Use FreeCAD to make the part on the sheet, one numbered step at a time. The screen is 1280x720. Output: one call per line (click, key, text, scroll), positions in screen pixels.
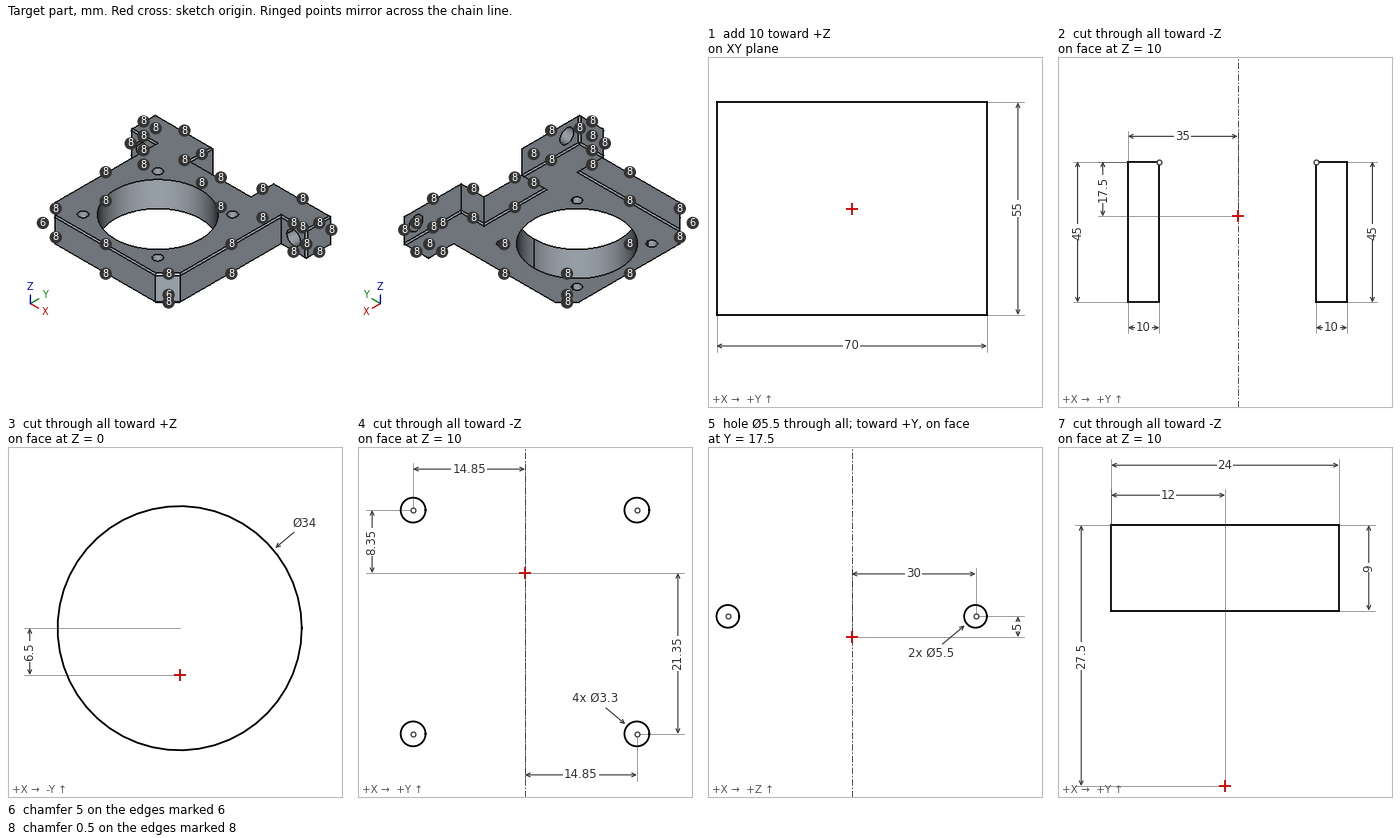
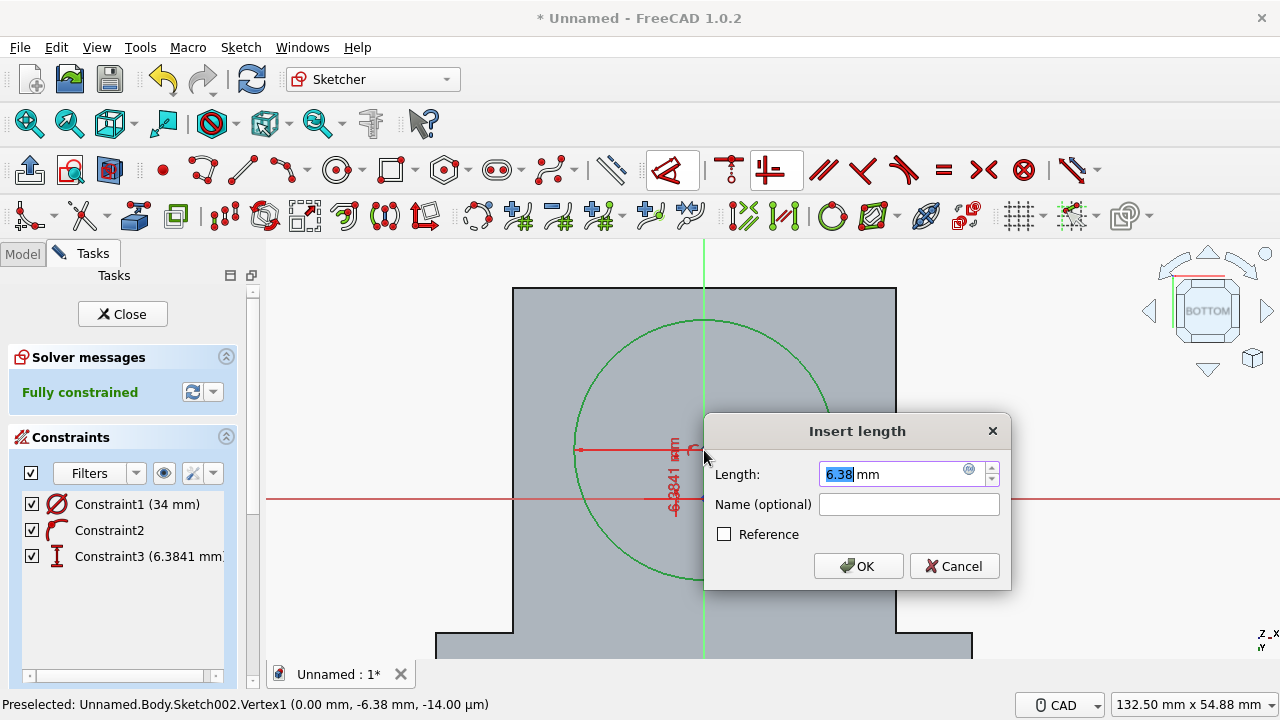
text(6.5)
key(Return)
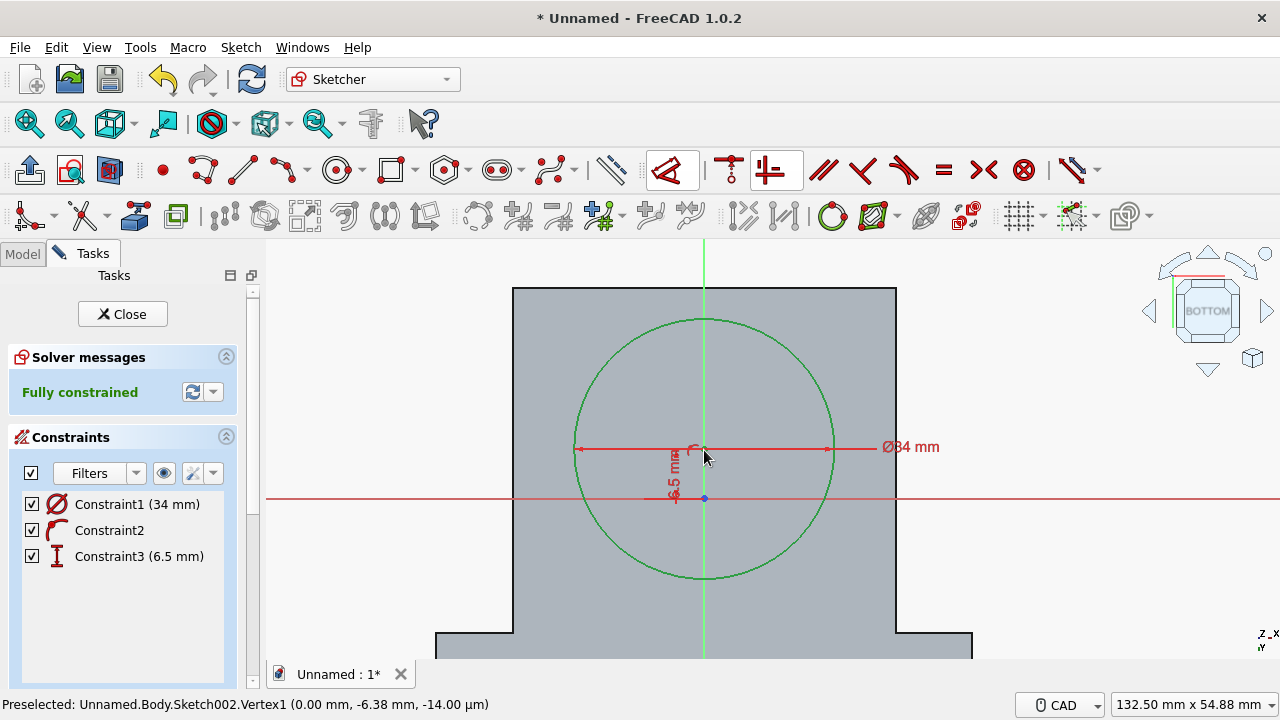
click(123, 314)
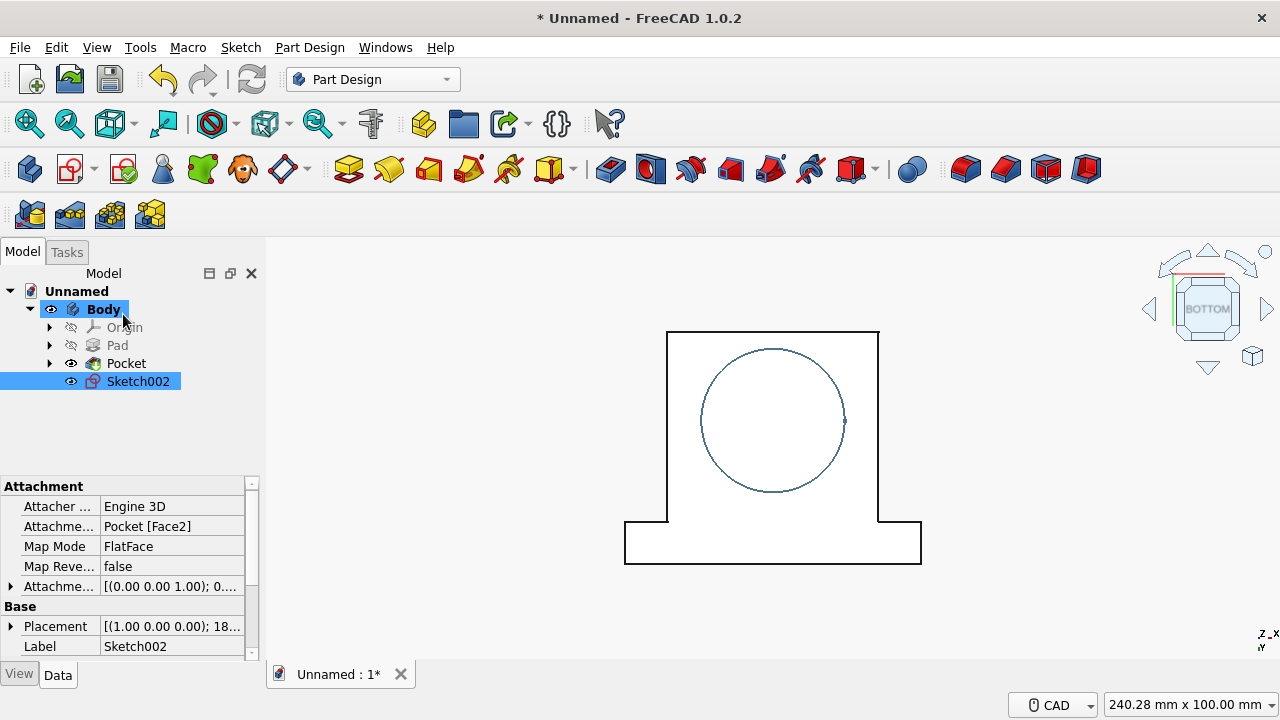
click(612, 170)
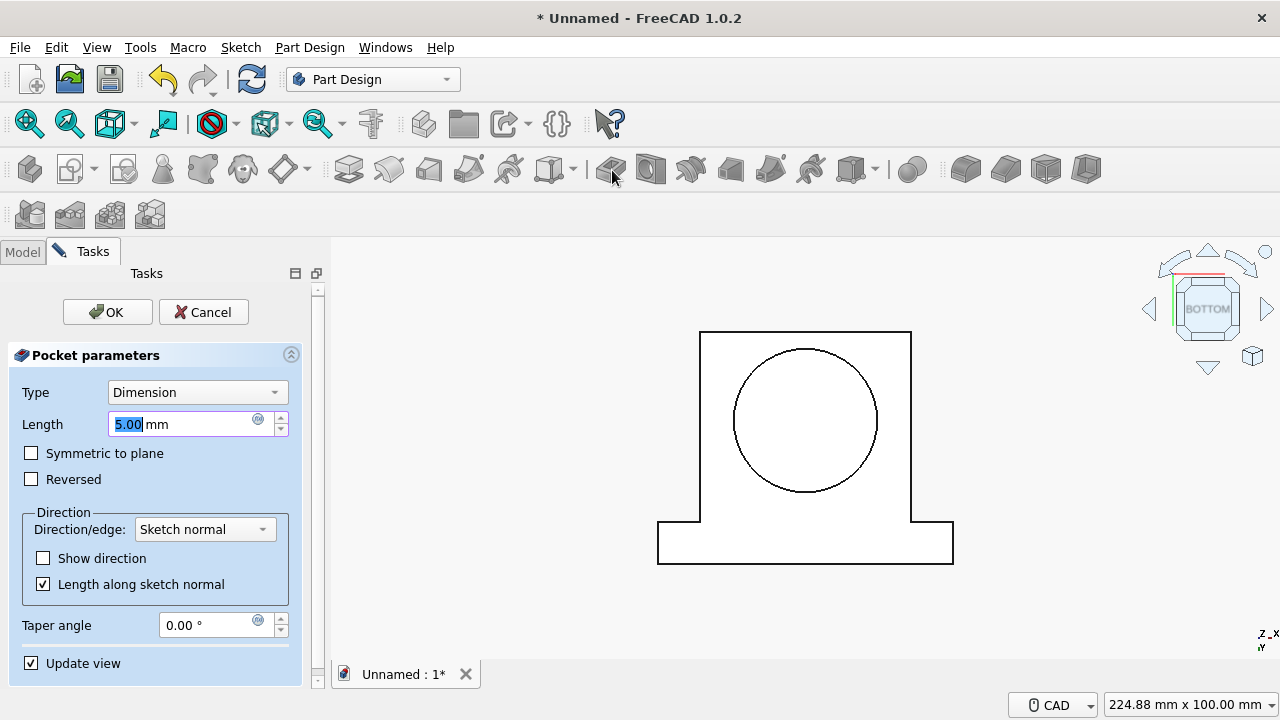
click(198, 392)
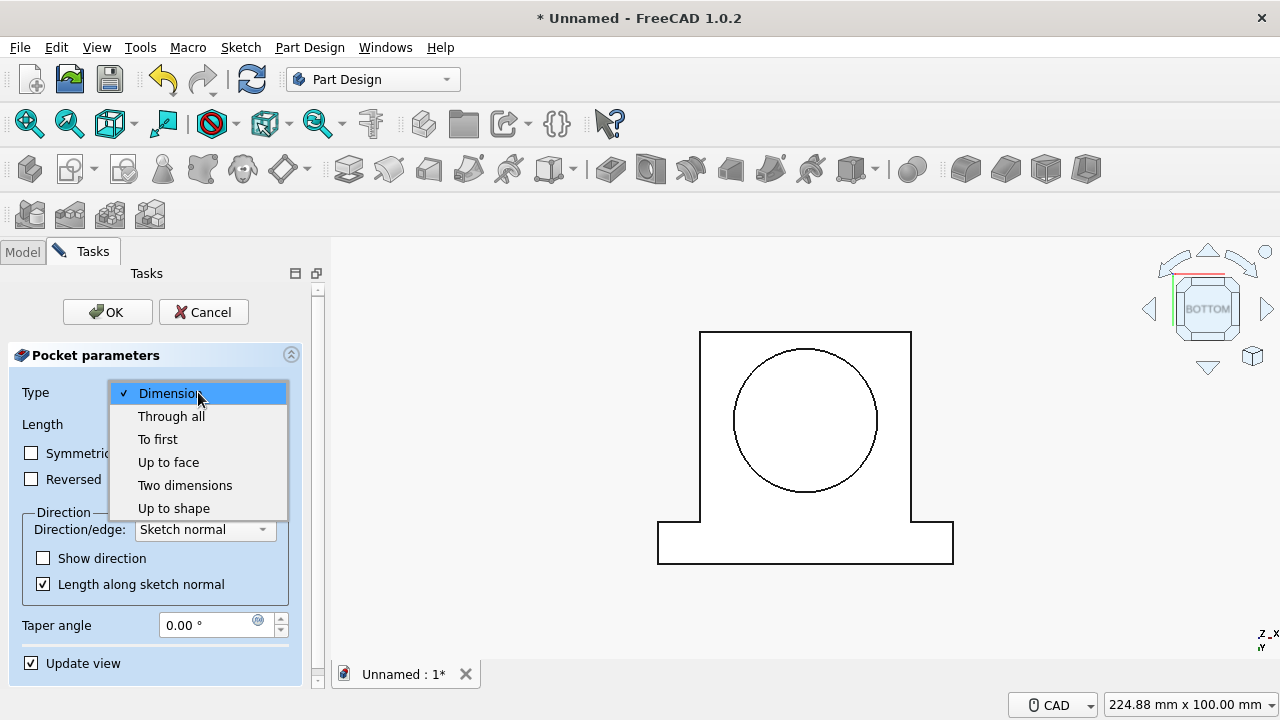
click(198, 416)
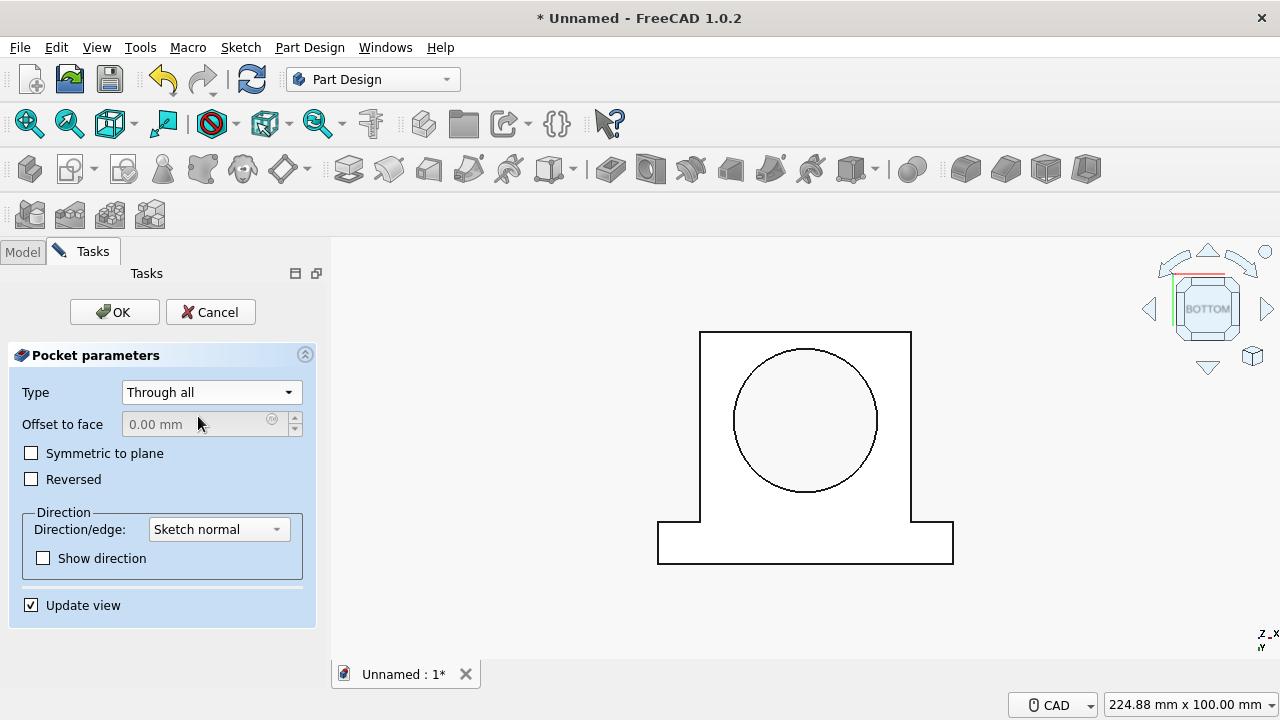
click(115, 312)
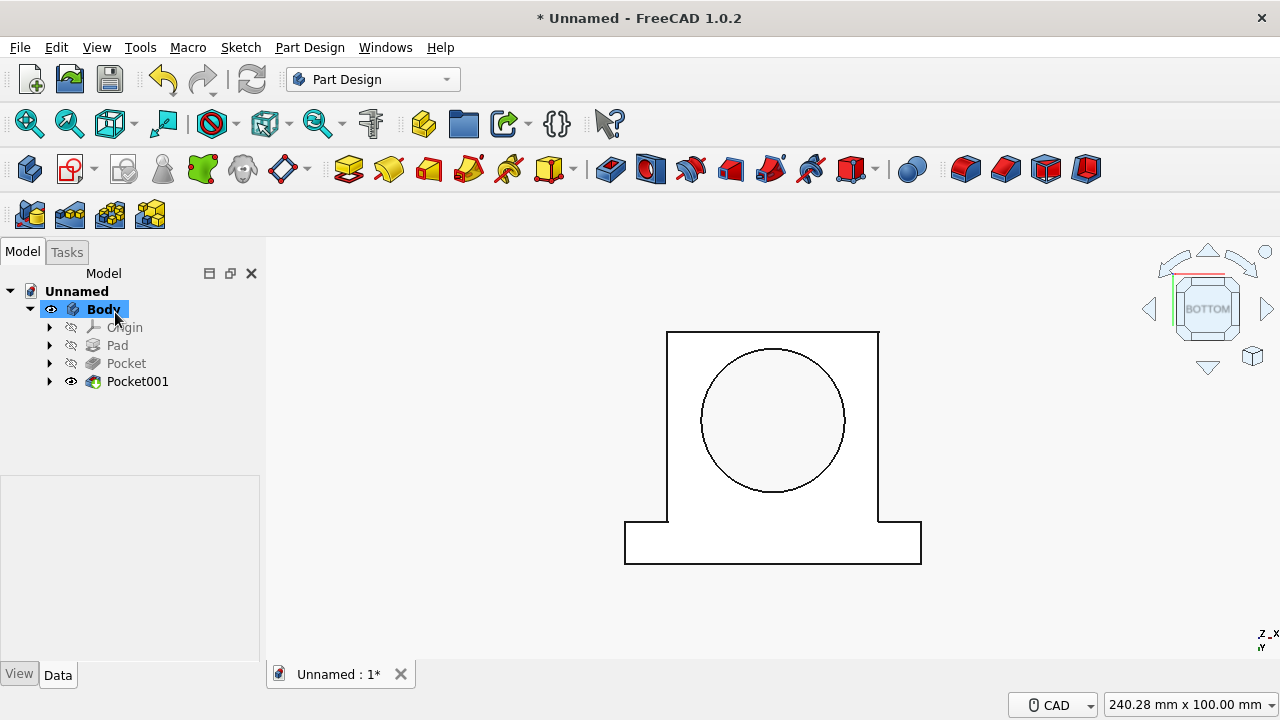
key(0)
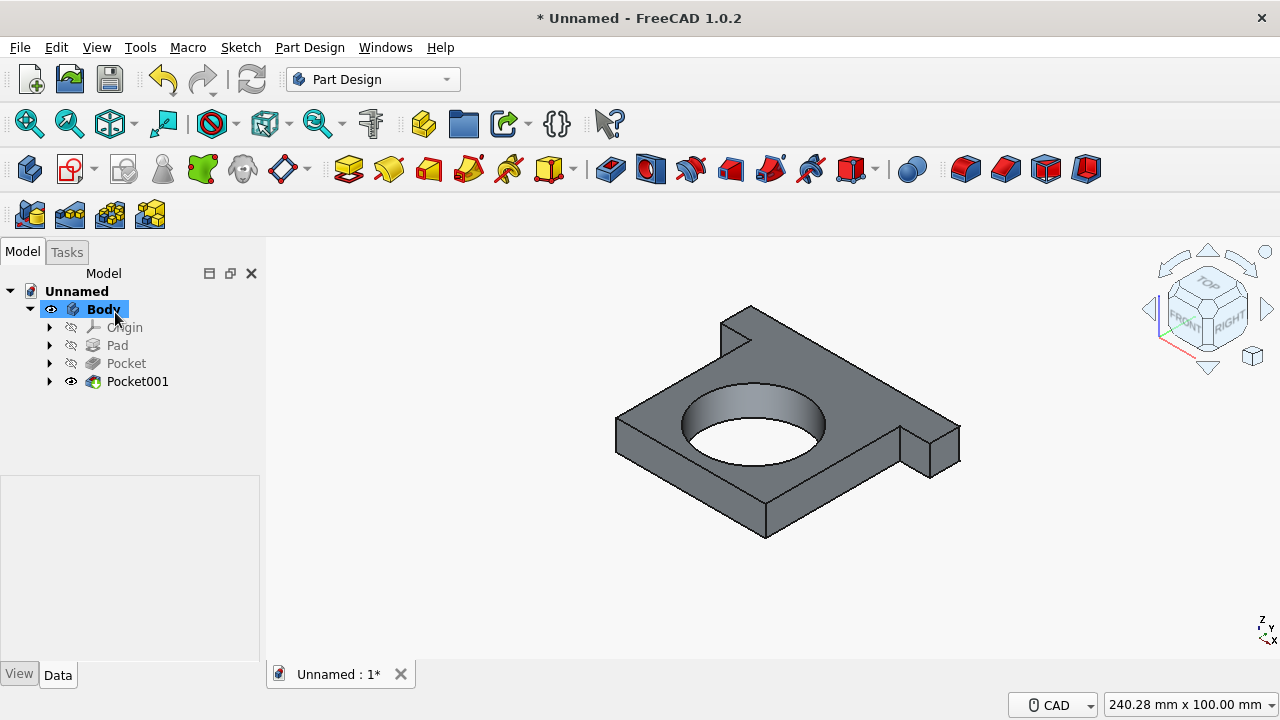
click(850, 403)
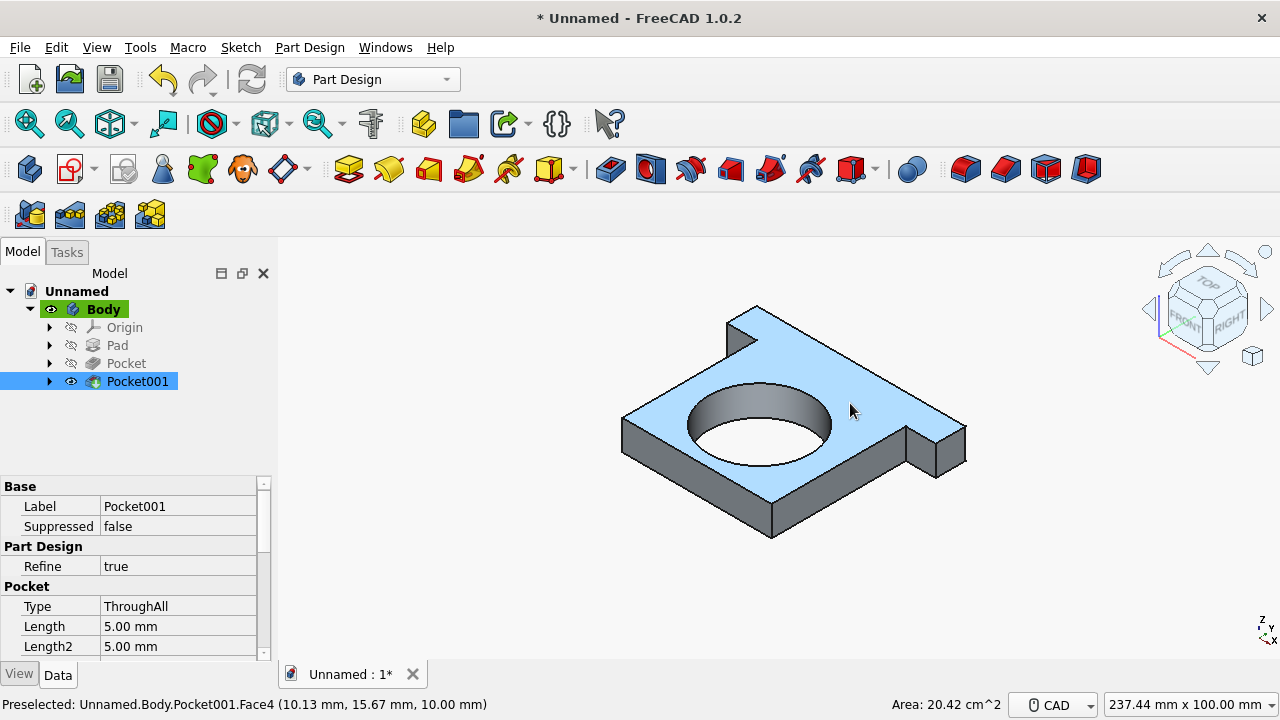
click(70, 170)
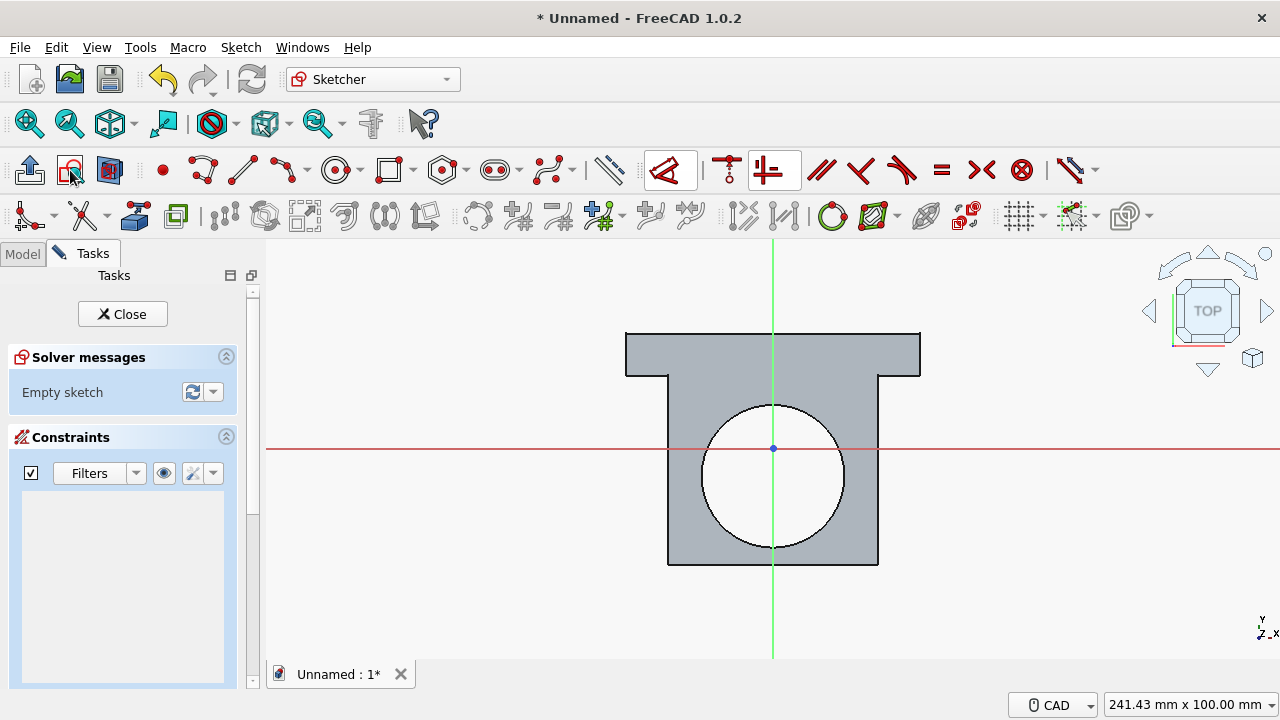
scroll(856, 510, up, 3)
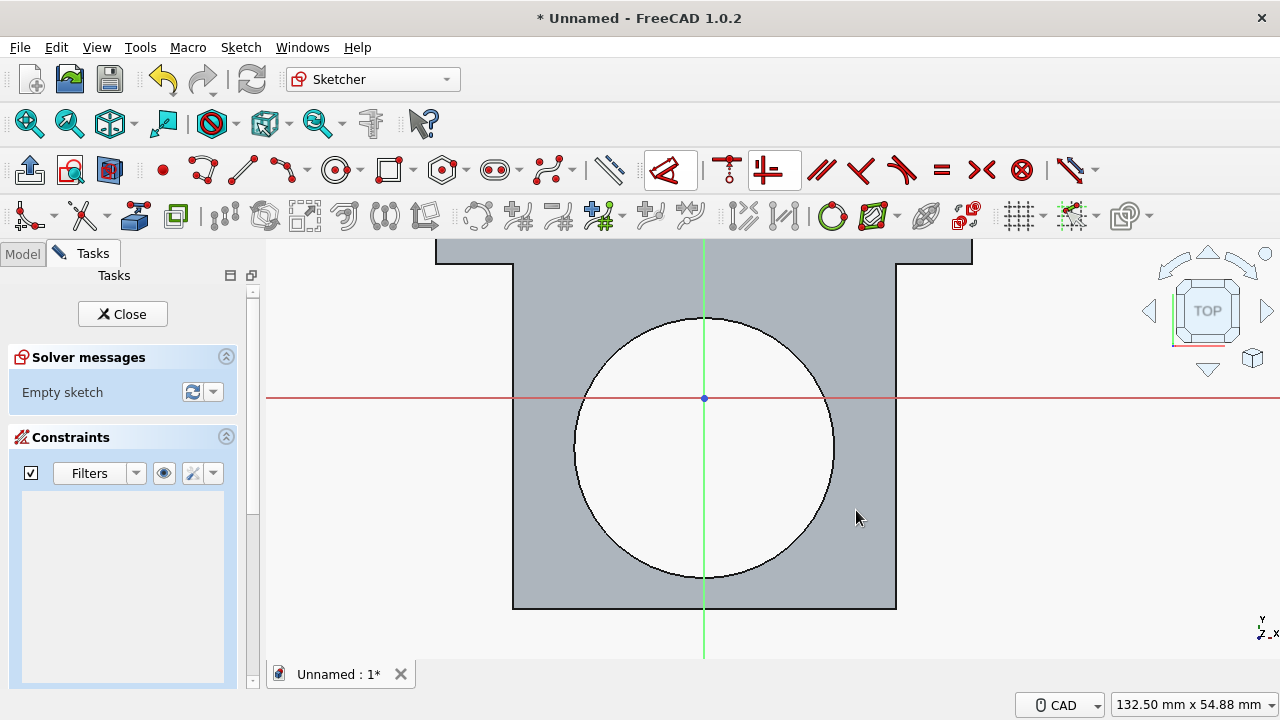
key(g)
key(c)